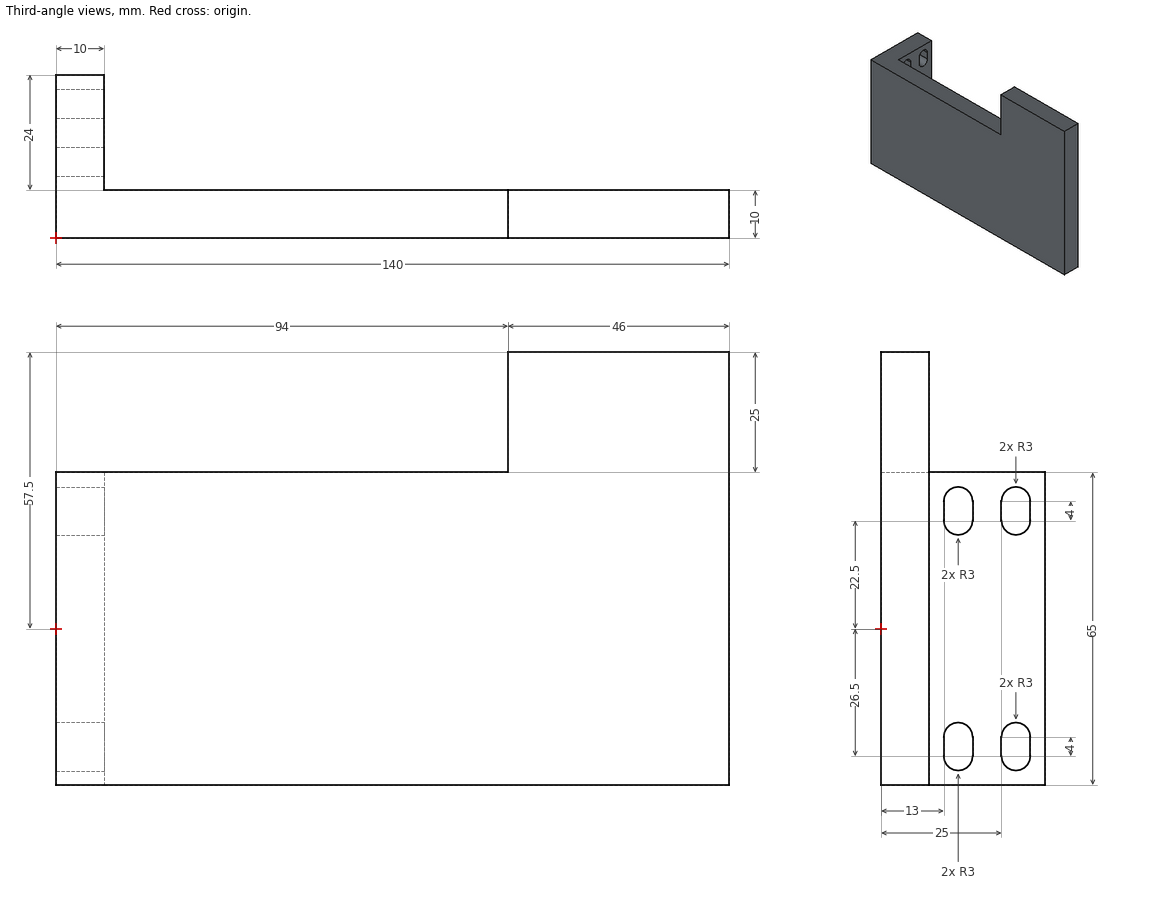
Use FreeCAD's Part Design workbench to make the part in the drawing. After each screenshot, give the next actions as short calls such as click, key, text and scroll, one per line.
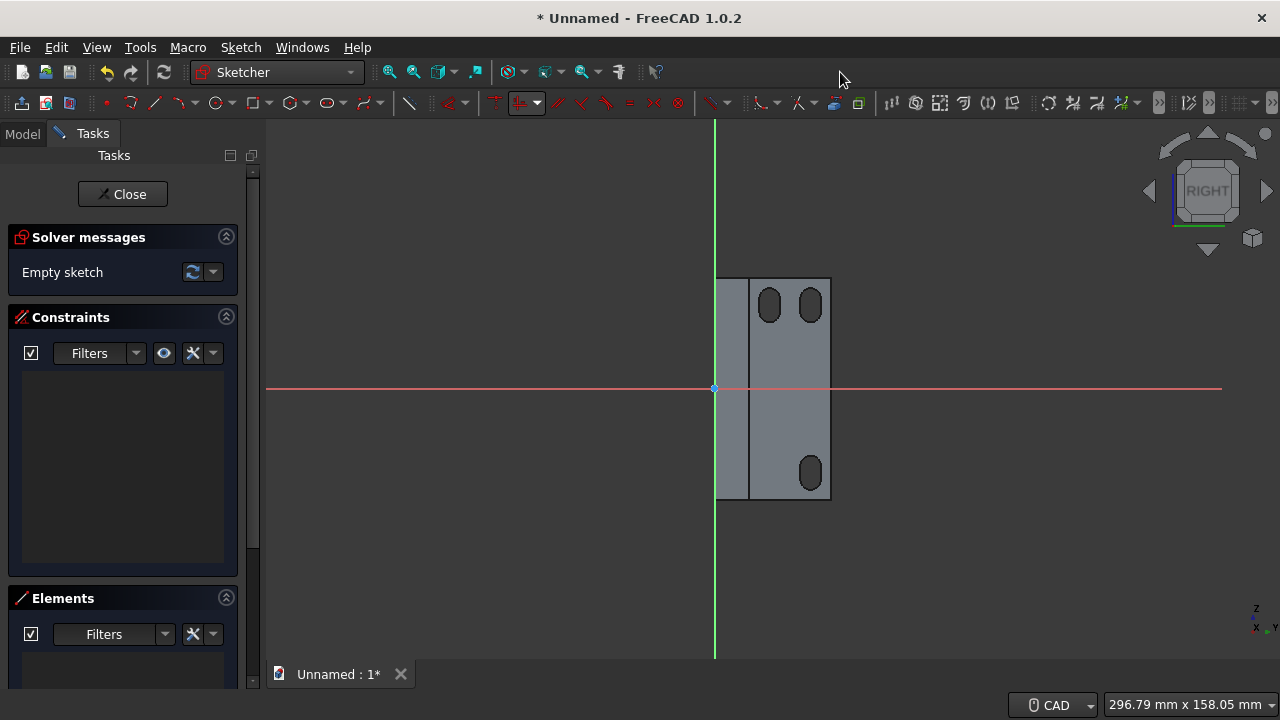
scroll(776, 481, up, 12)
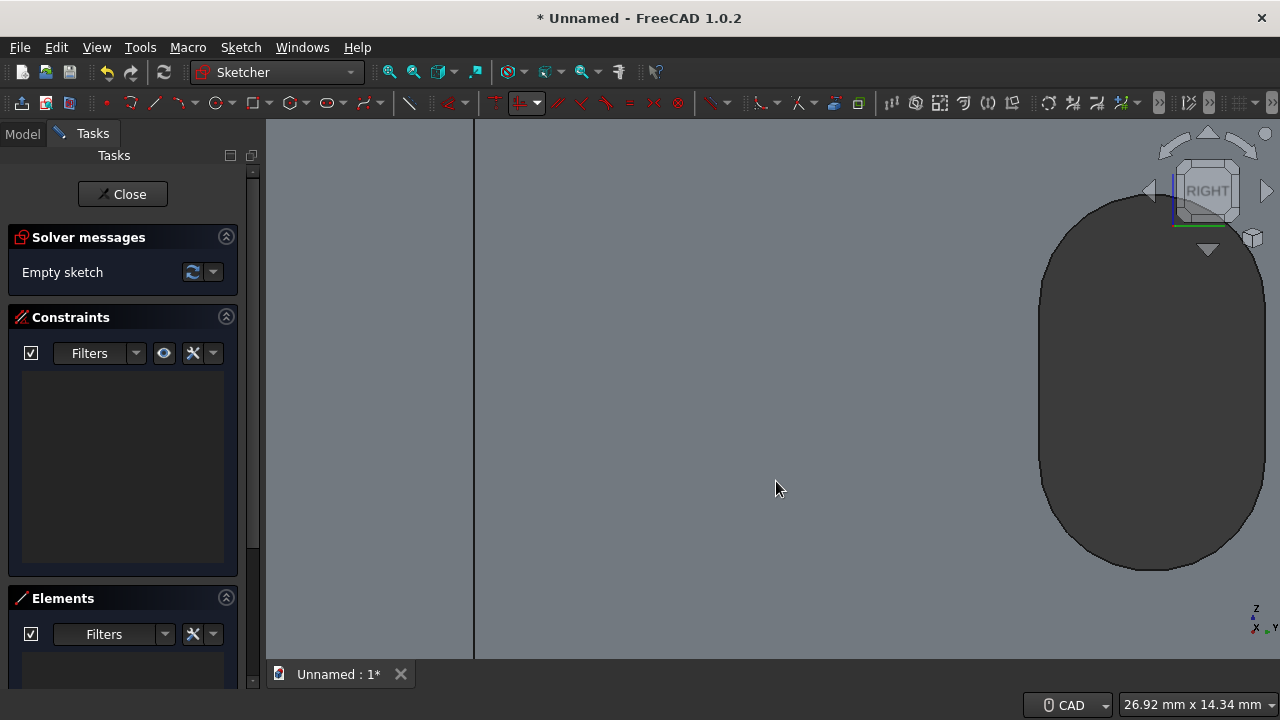
click(328, 104)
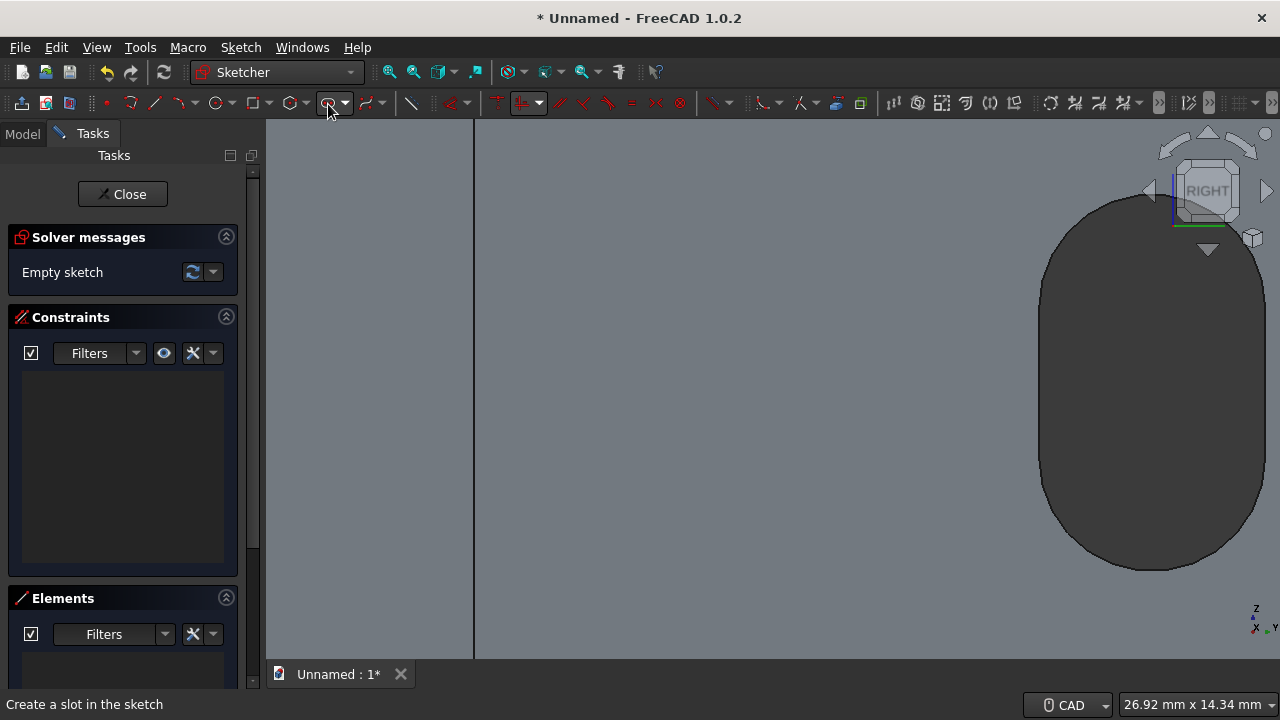
click(700, 458)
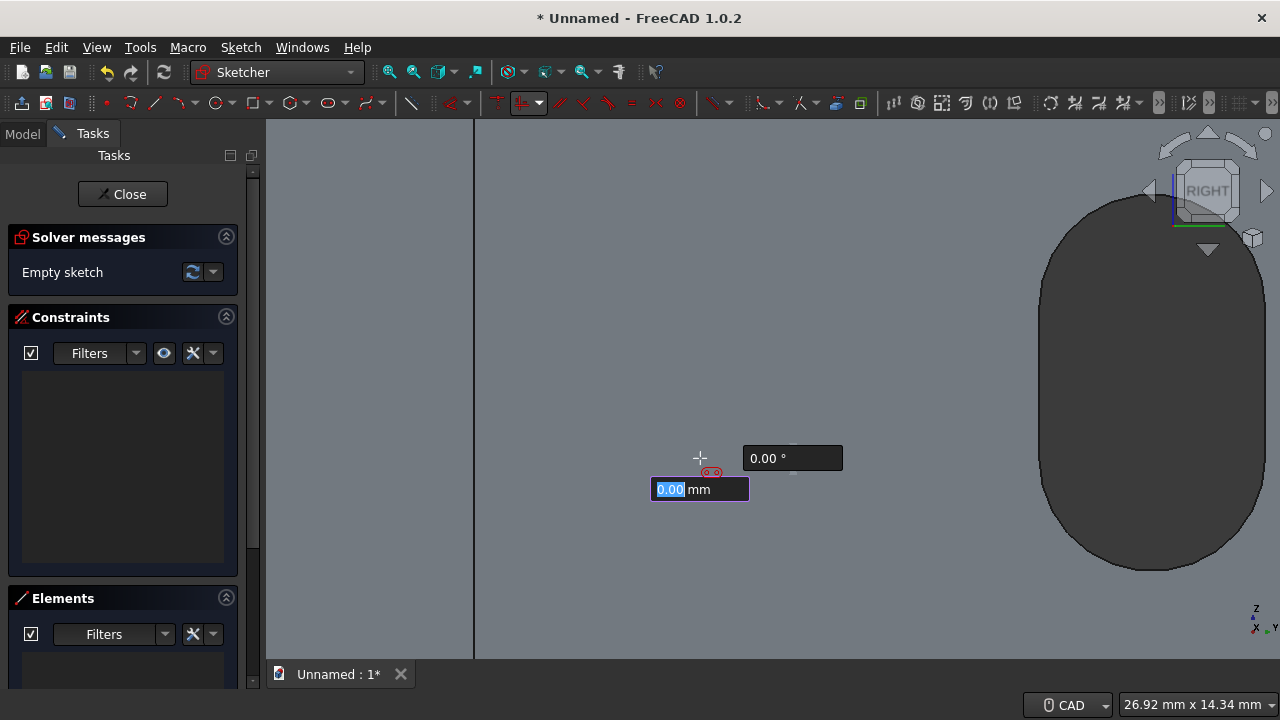
click(700, 308)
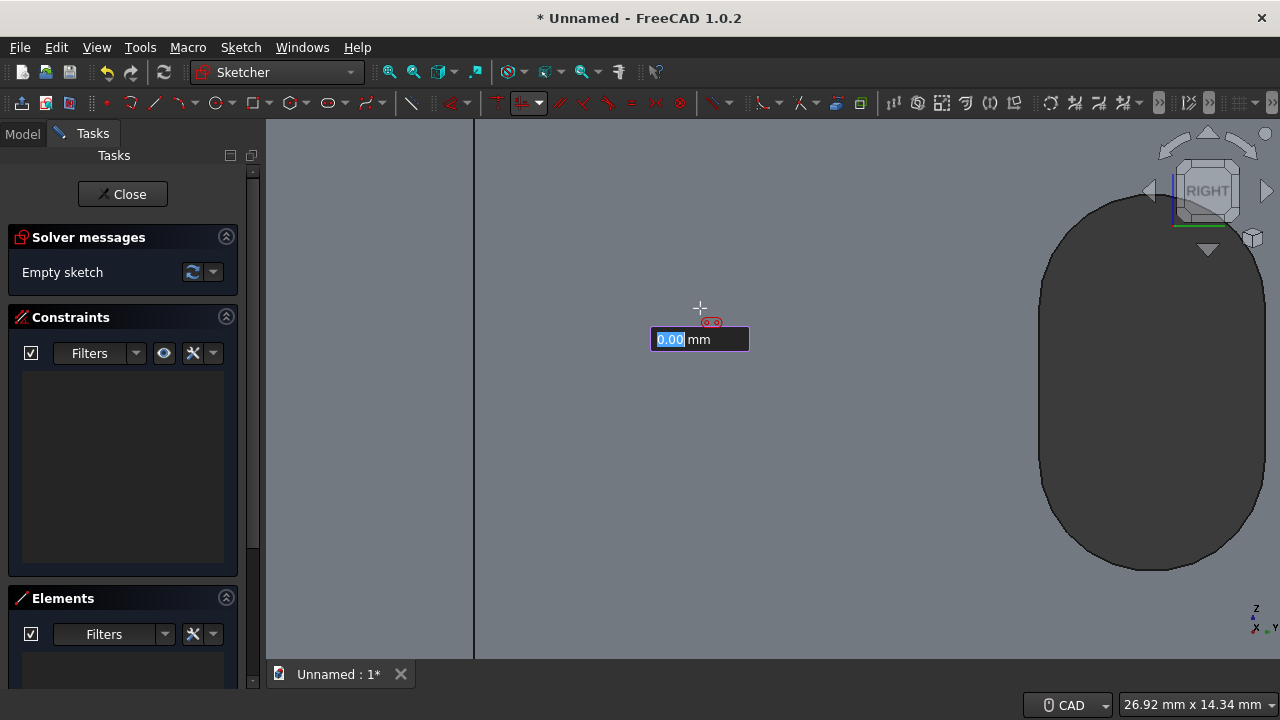
click(587, 383)
key(Escape)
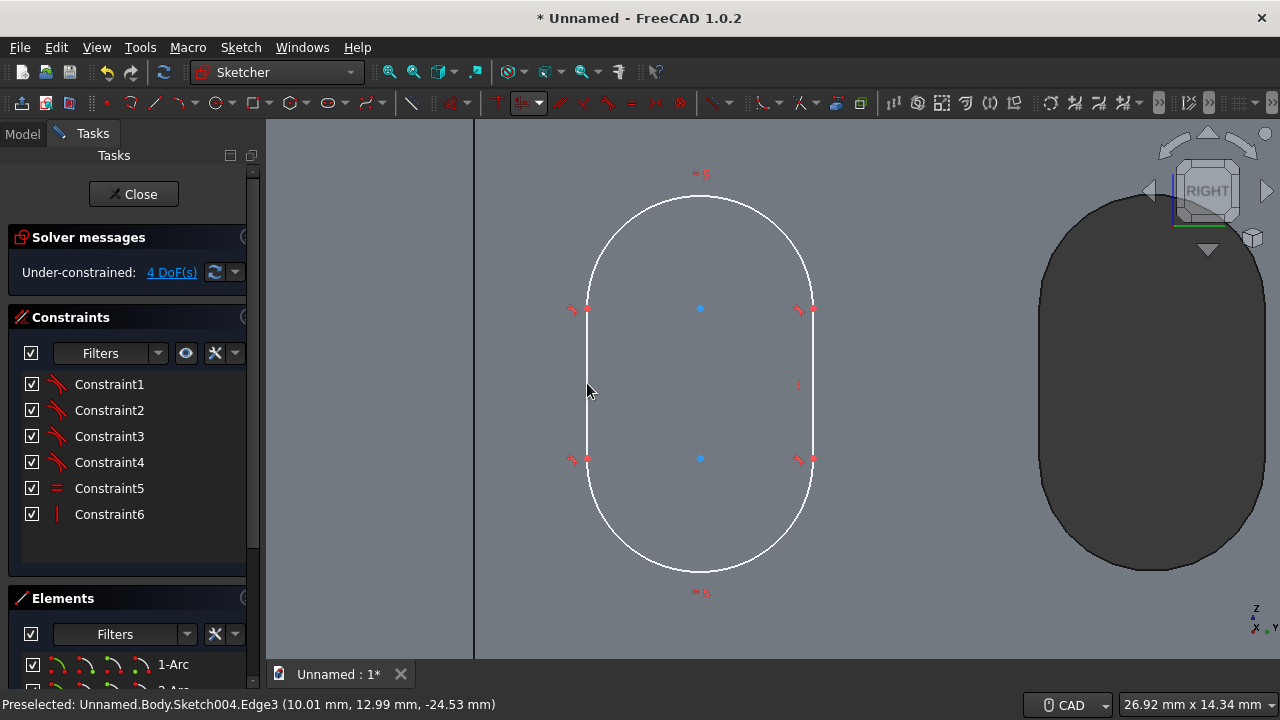
key(d)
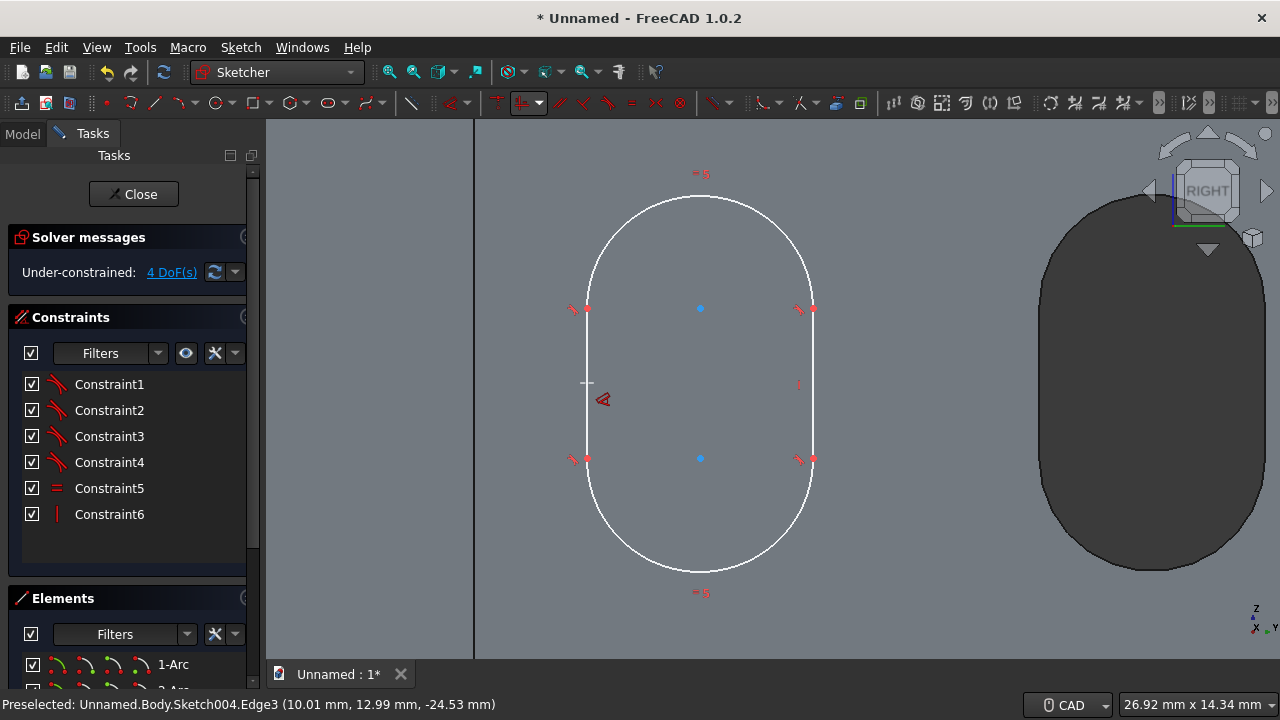
click(634, 550)
click(615, 576)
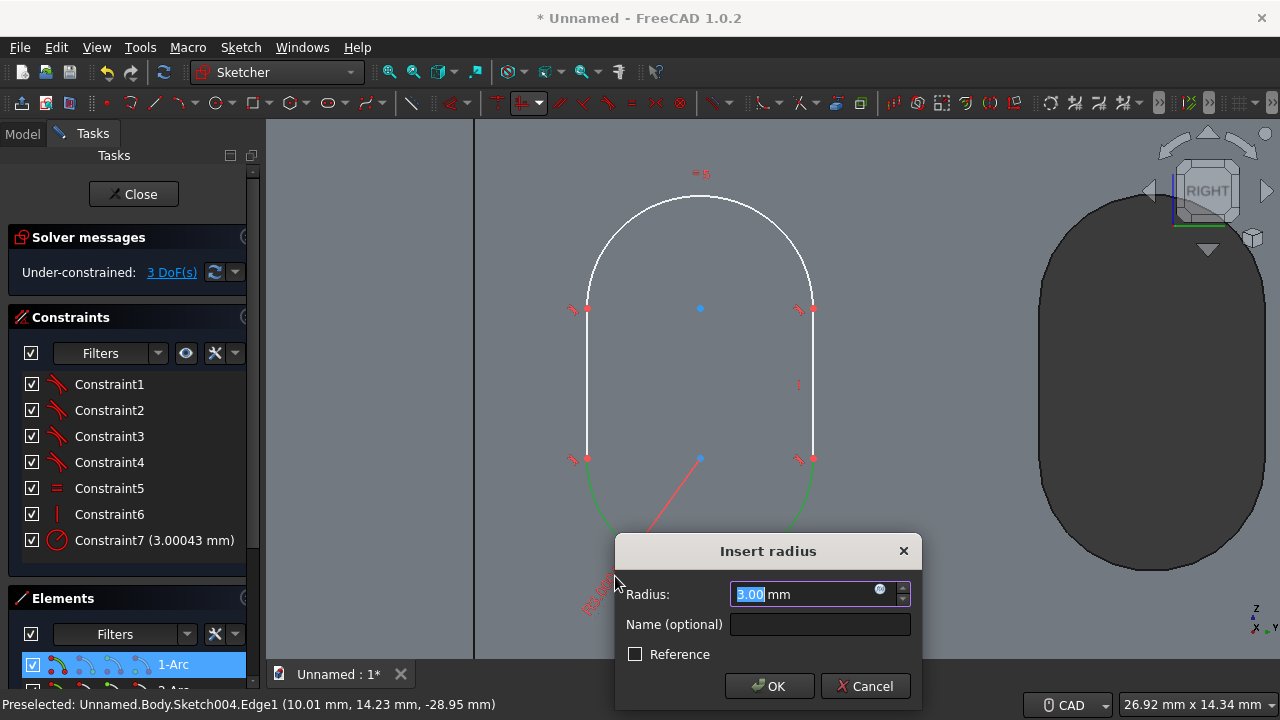
text(3)
key(Return)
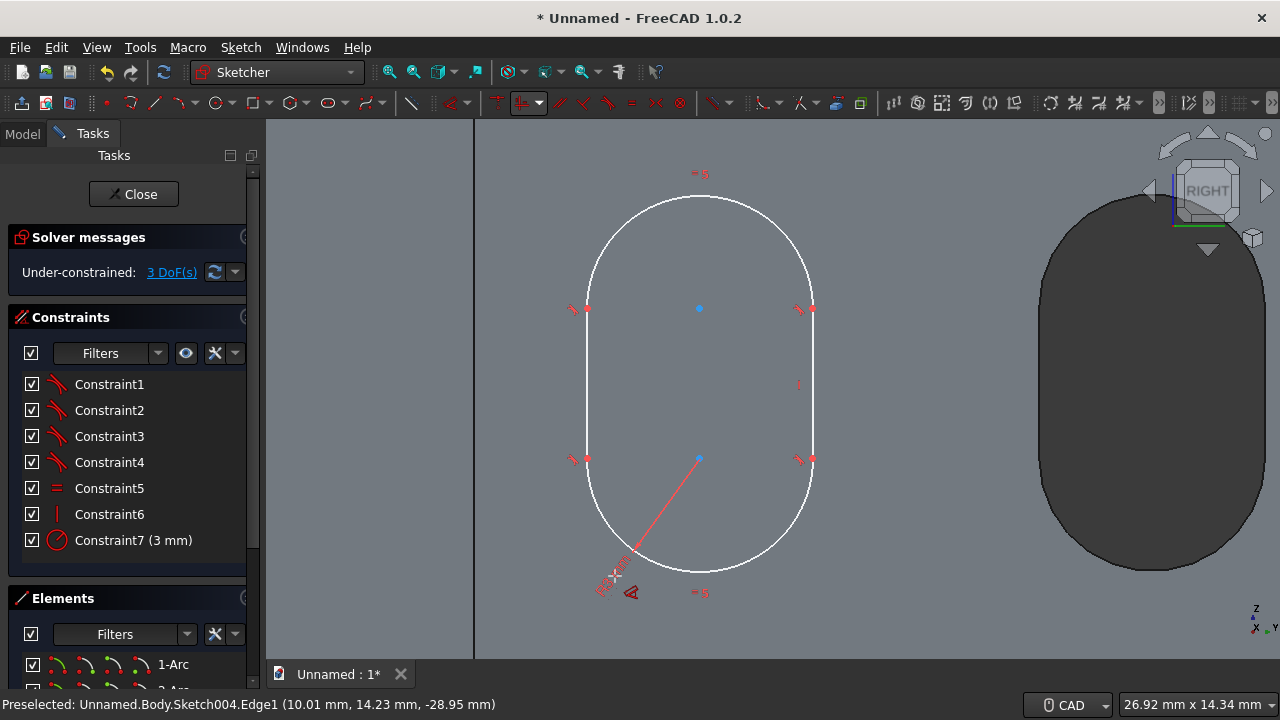
click(587, 414)
click(553, 384)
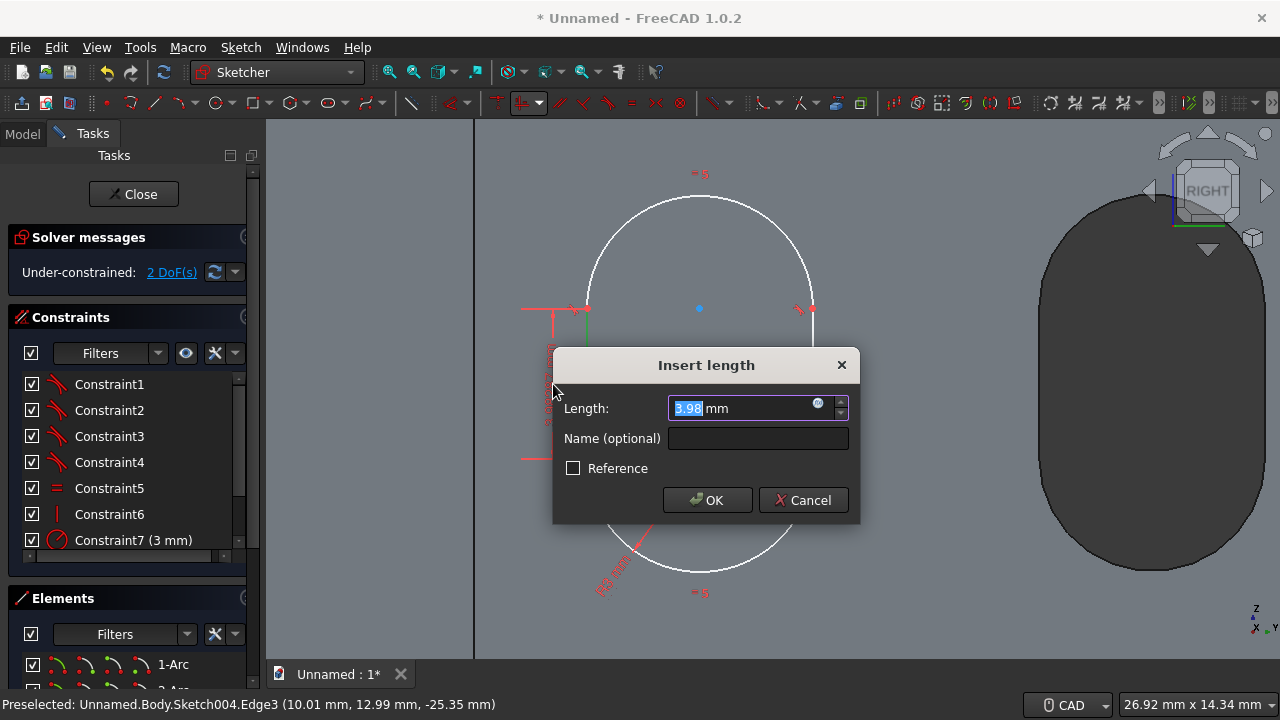
text(4)
key(Return)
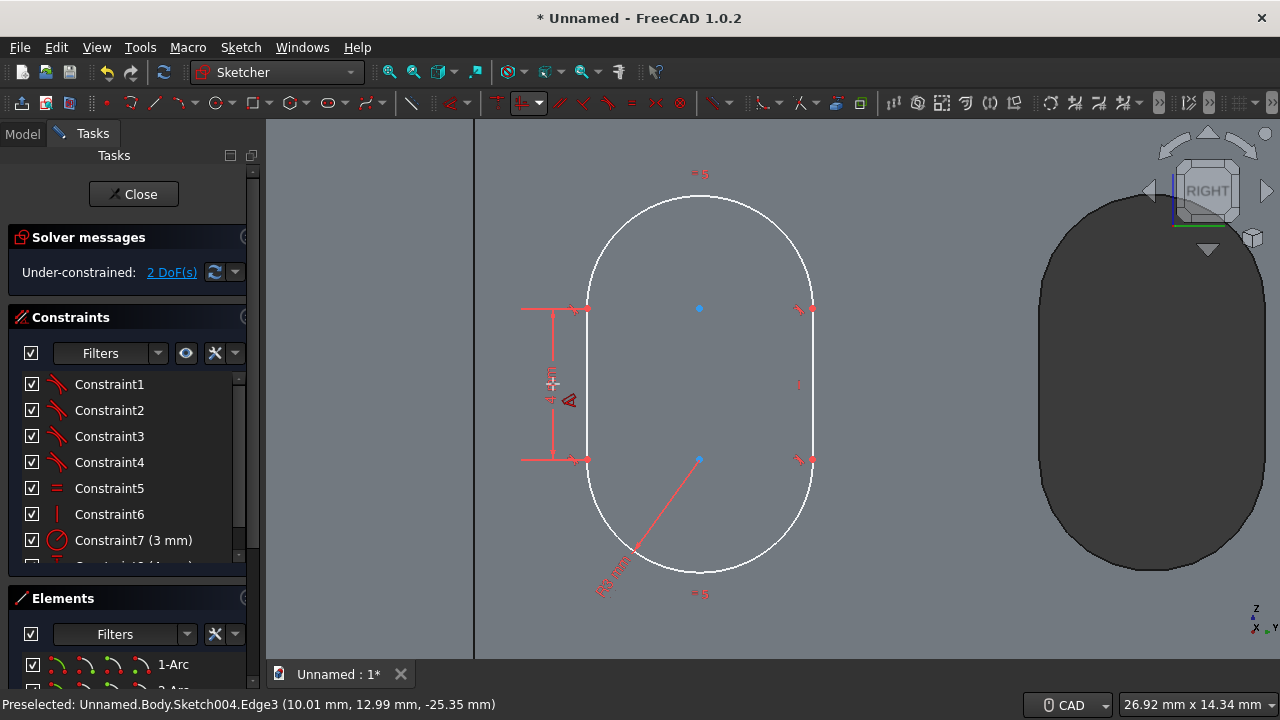
click(587, 460)
click(441, 494)